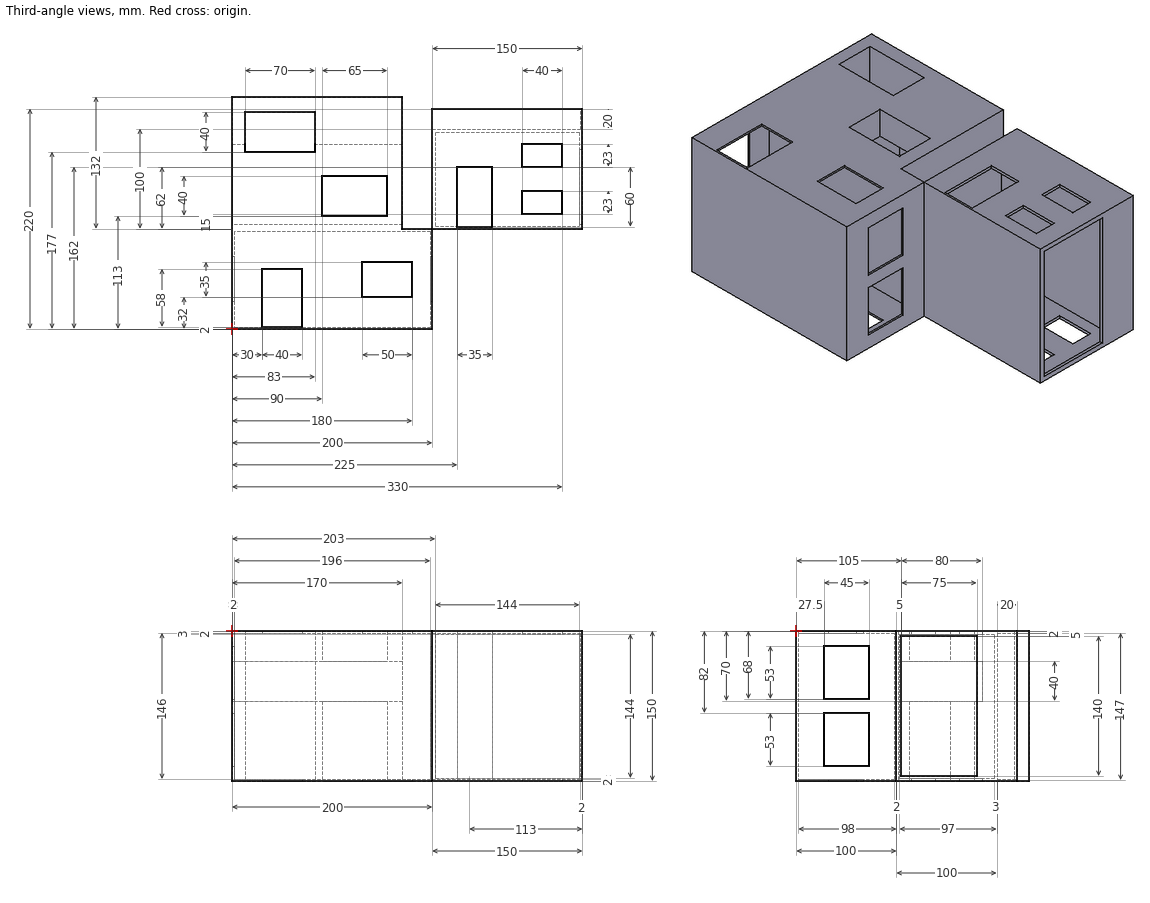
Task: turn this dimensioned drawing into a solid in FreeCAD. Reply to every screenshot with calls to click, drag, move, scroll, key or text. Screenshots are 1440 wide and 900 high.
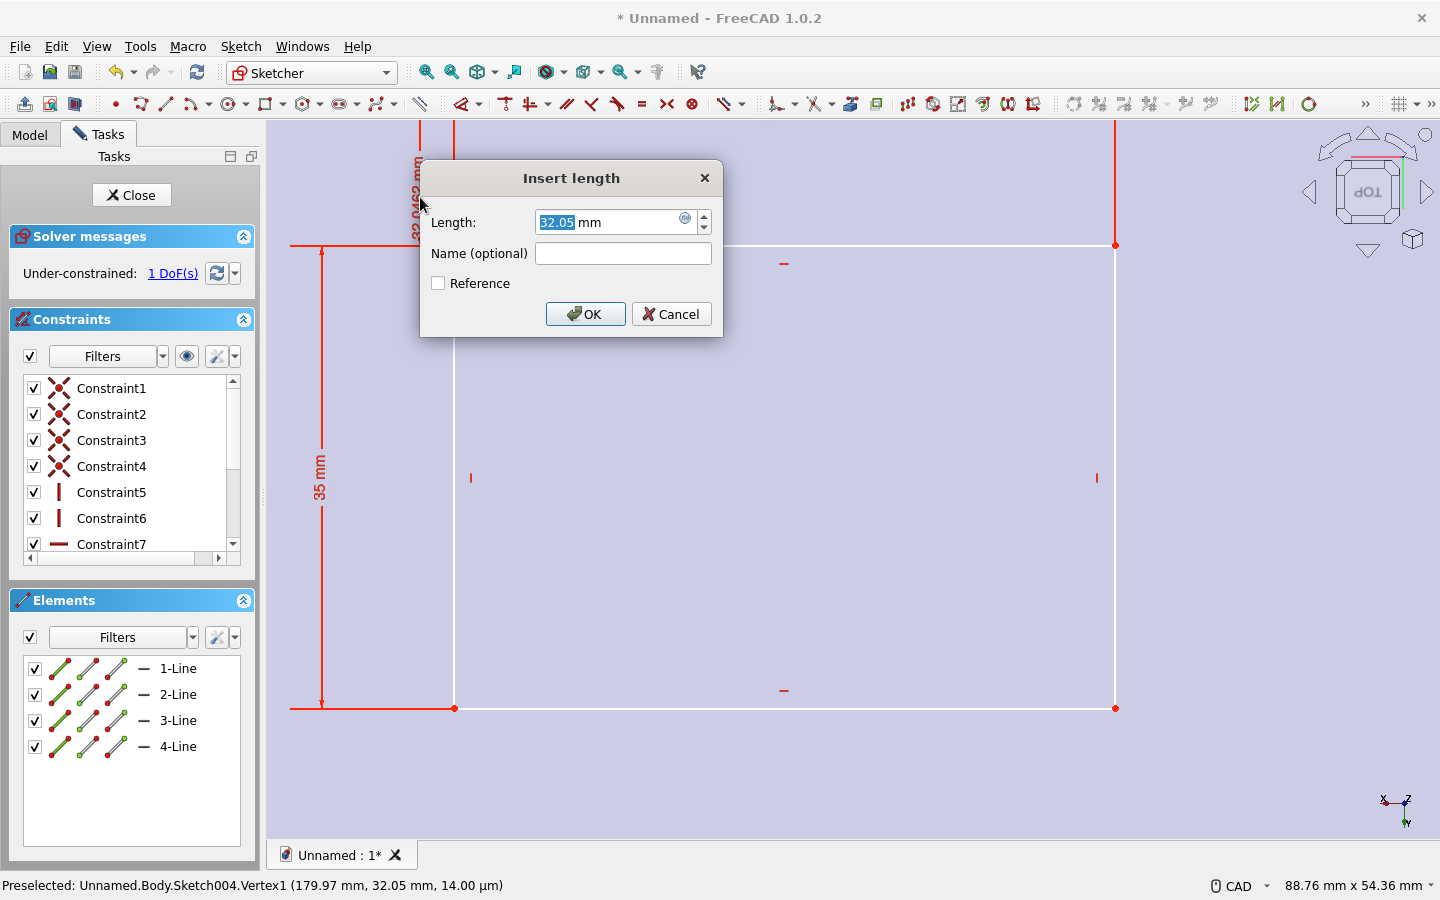
text(32)
key(Return)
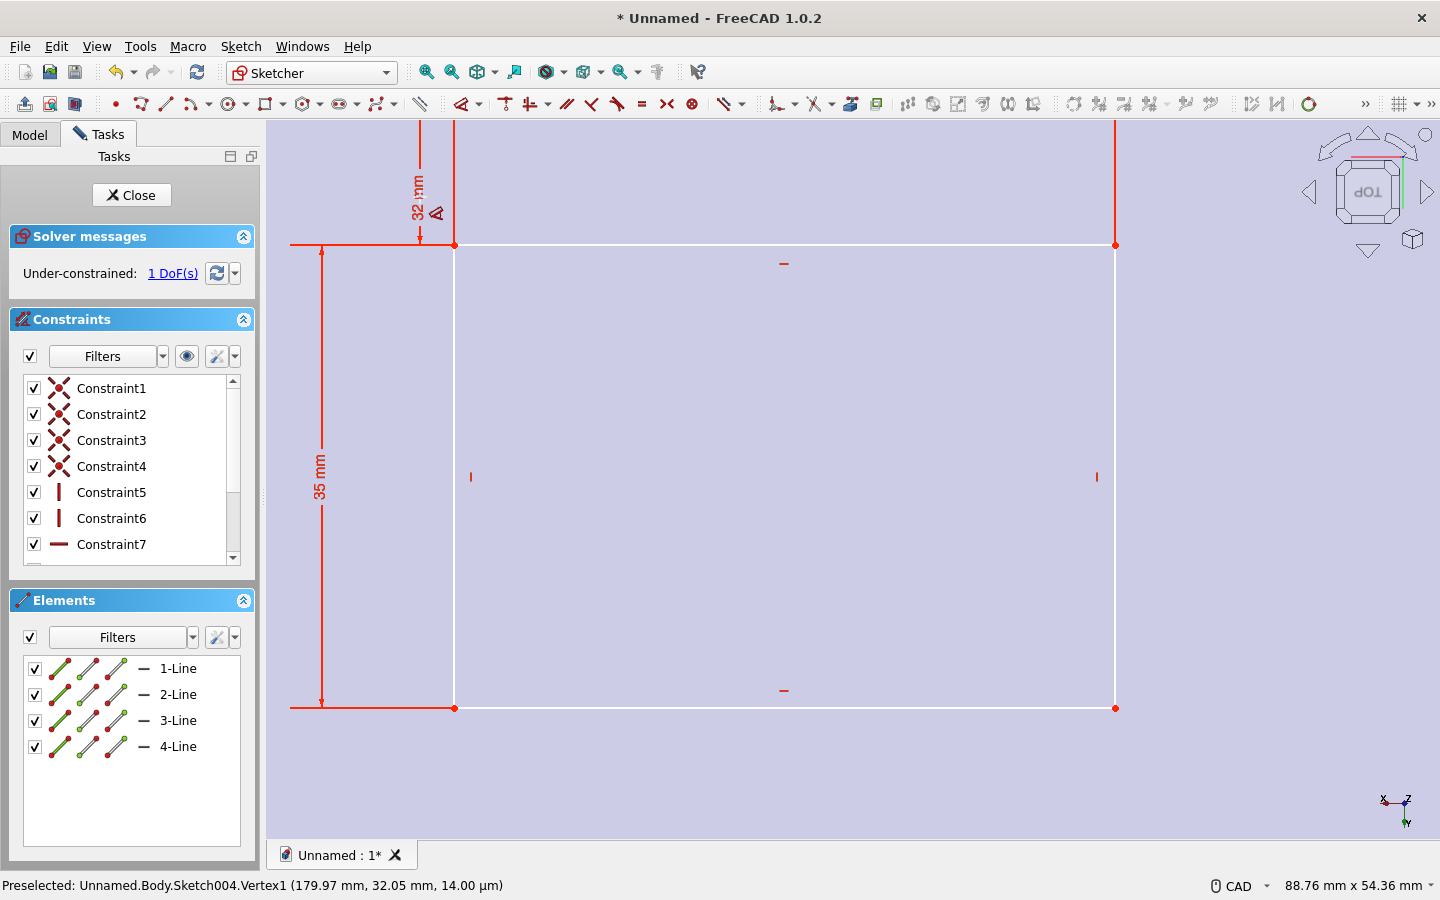
click(454, 245)
click(865, 279)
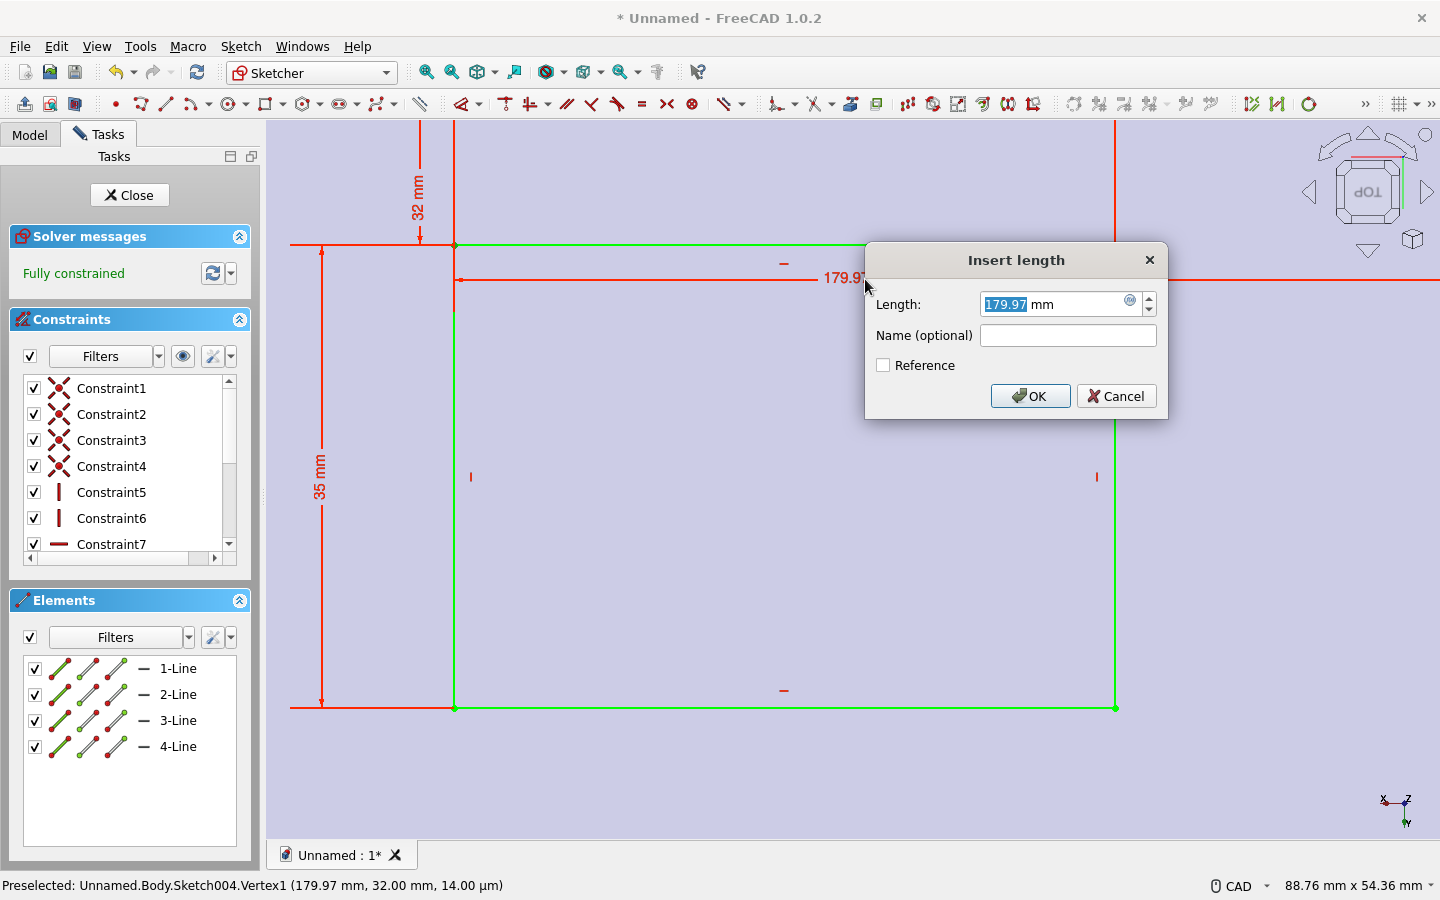
text(180)
key(Return)
key(Escape)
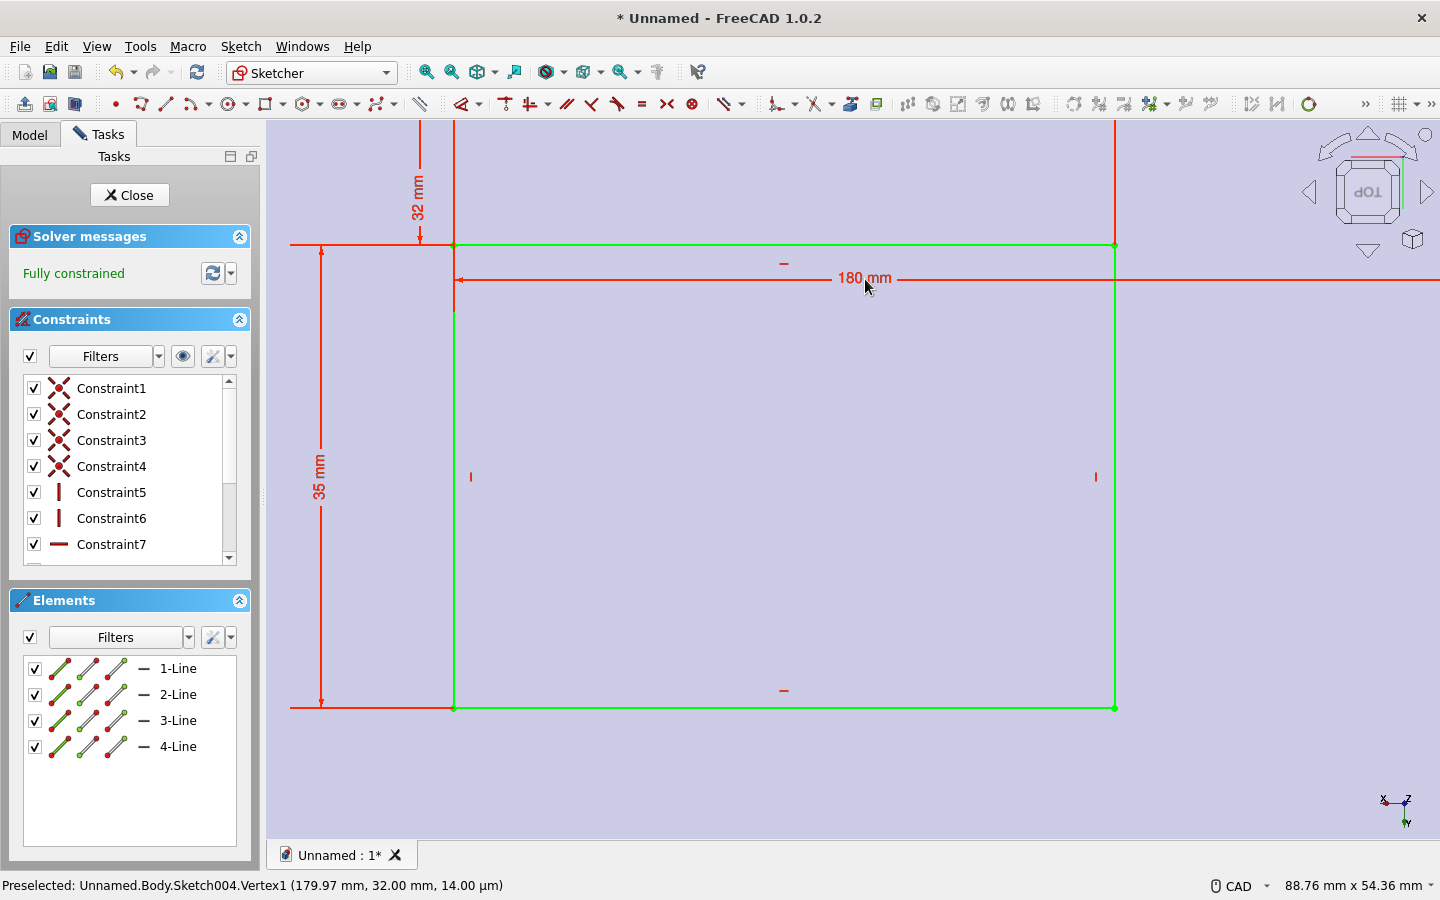
click(130, 195)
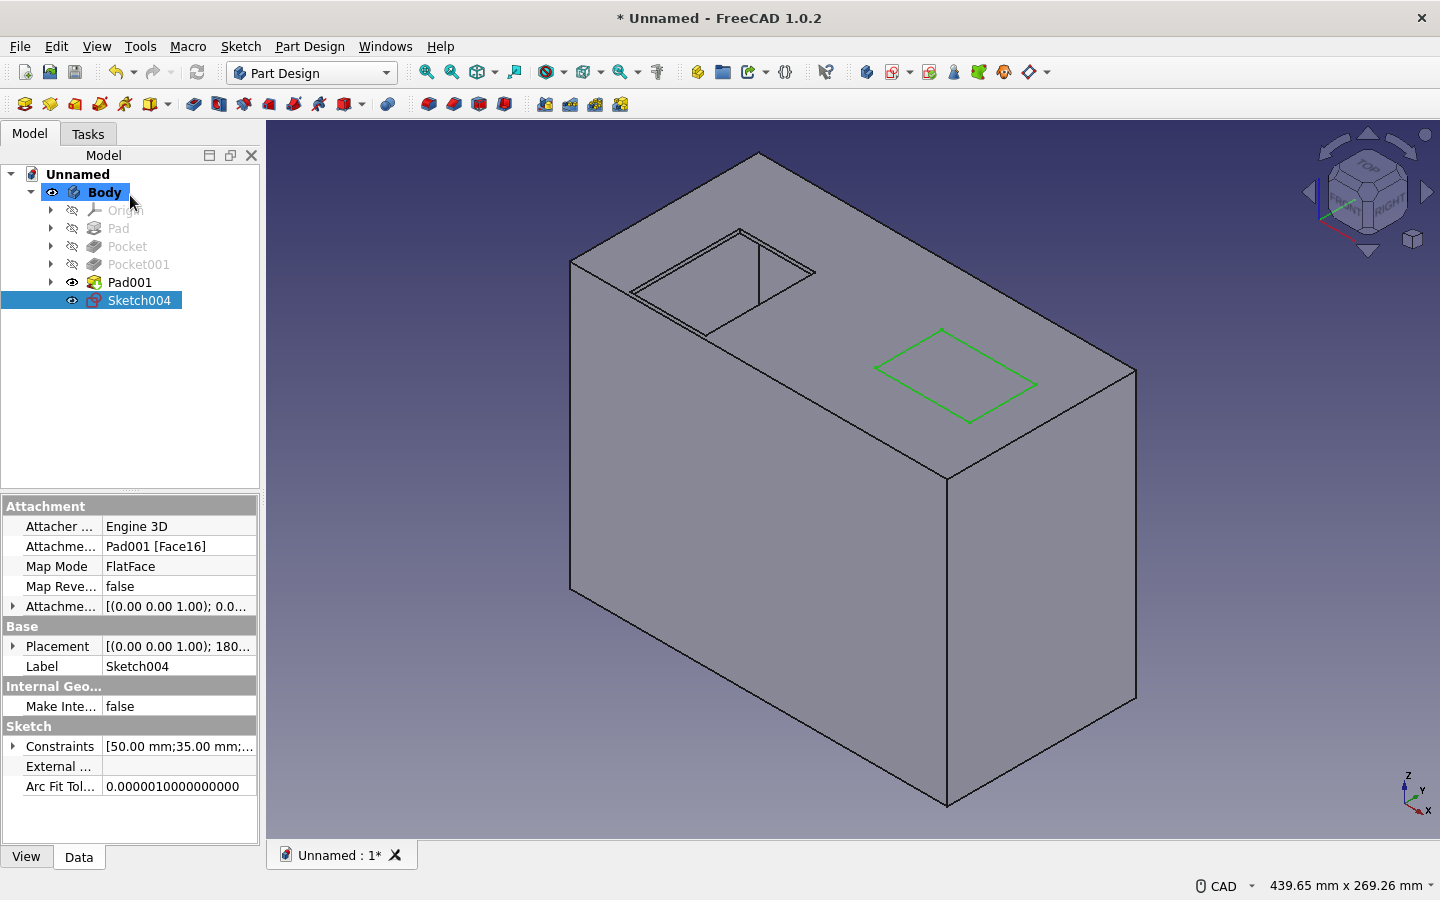
click(194, 104)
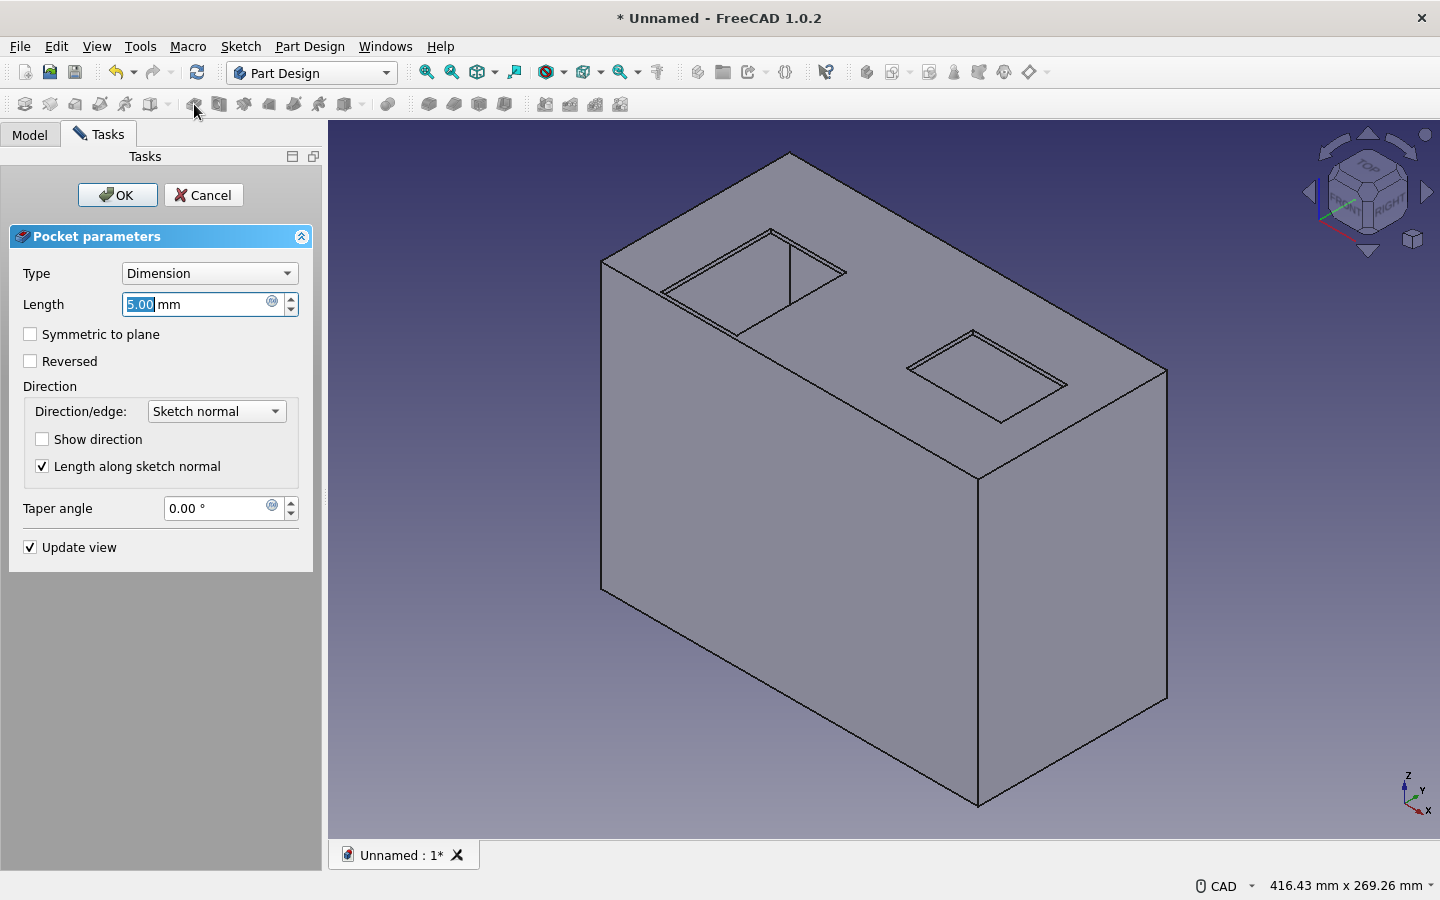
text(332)
key(Tab)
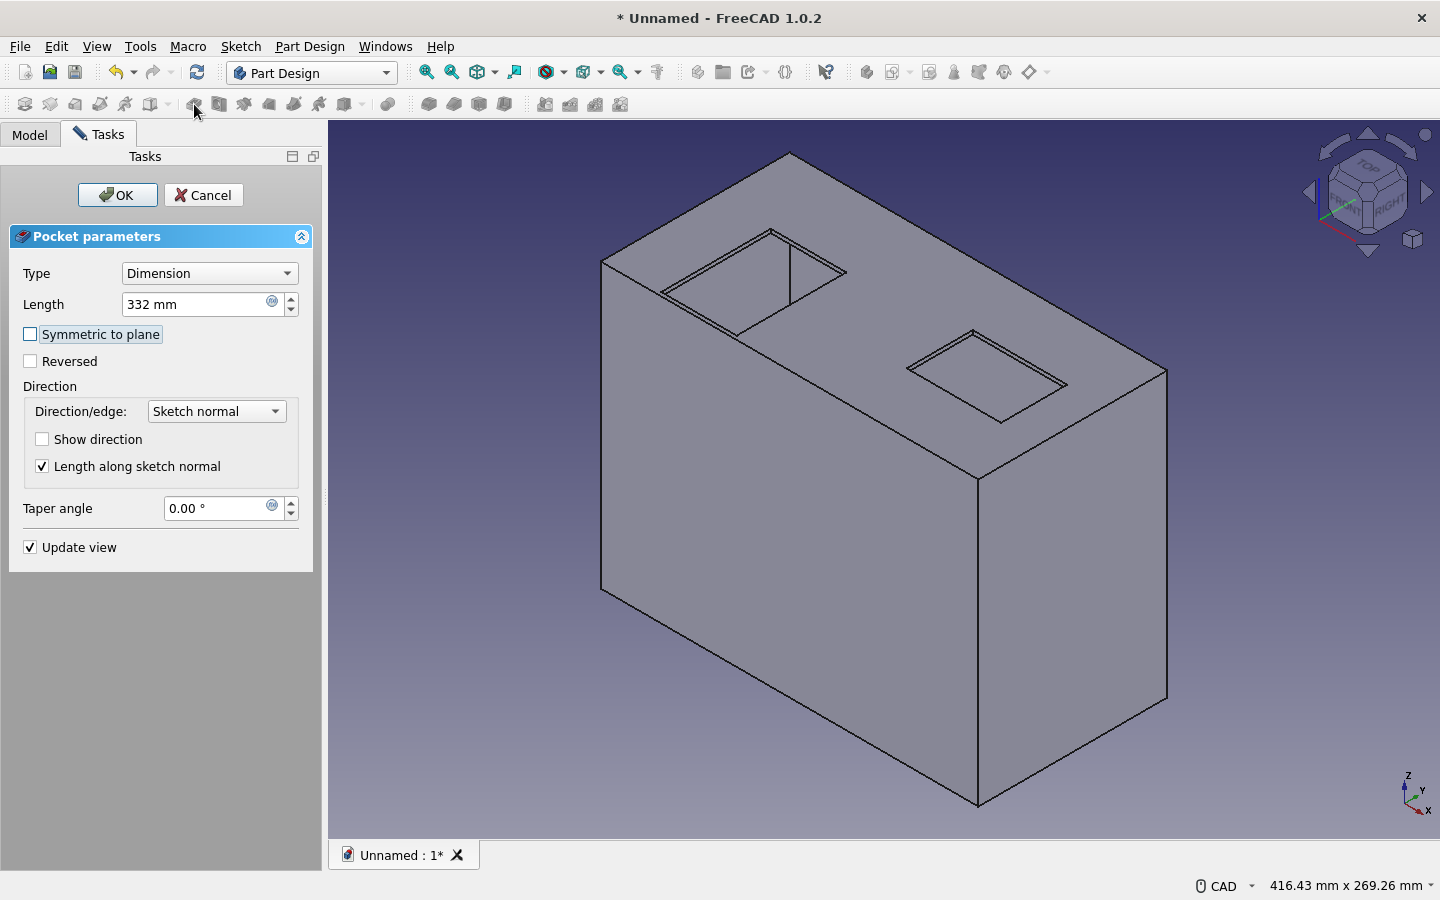
click(118, 195)